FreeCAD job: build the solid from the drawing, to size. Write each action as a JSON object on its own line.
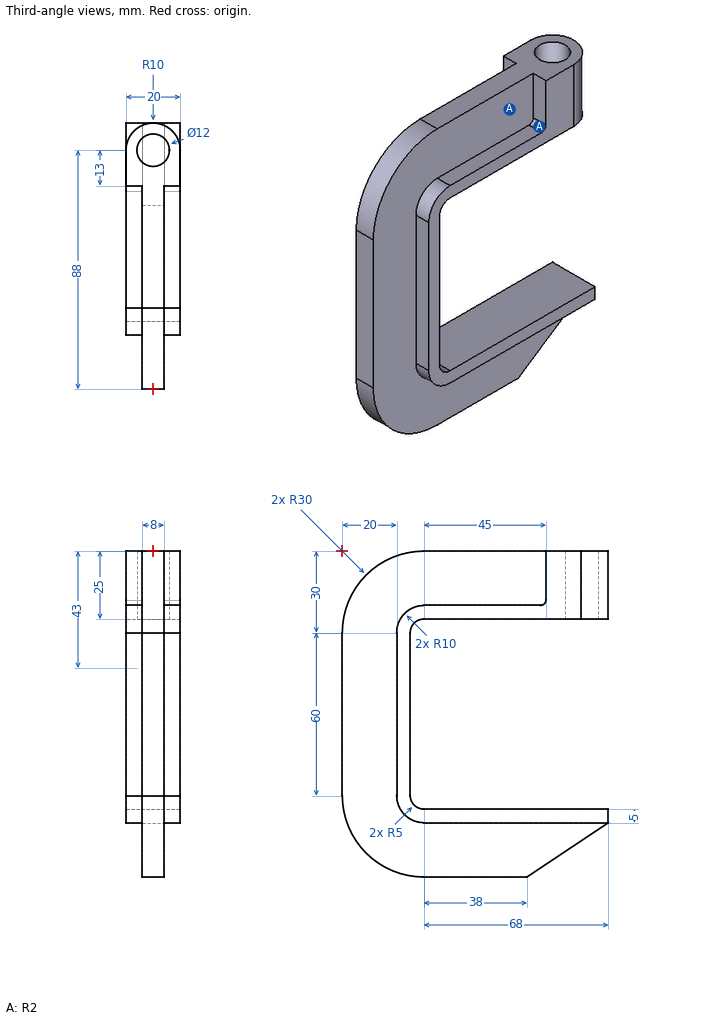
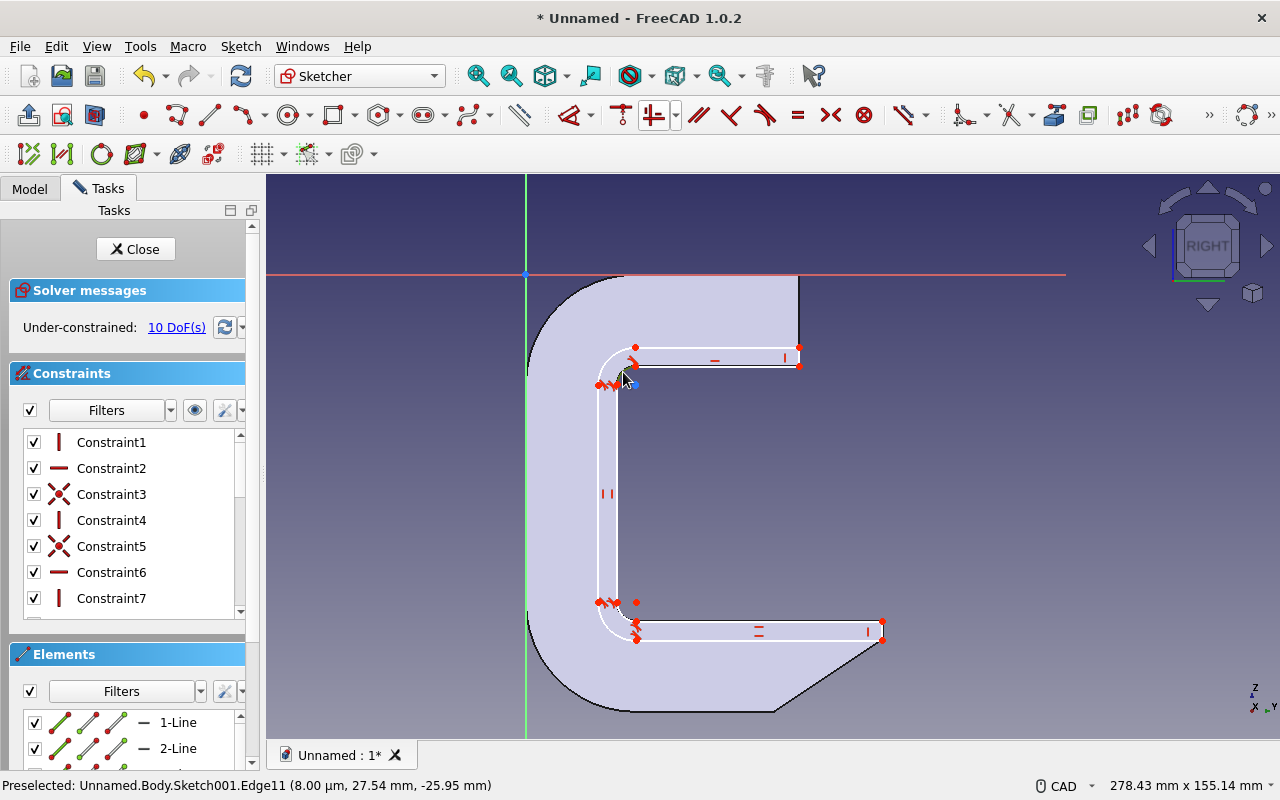
{"action": "left_click", "coordinate": [619, 352]}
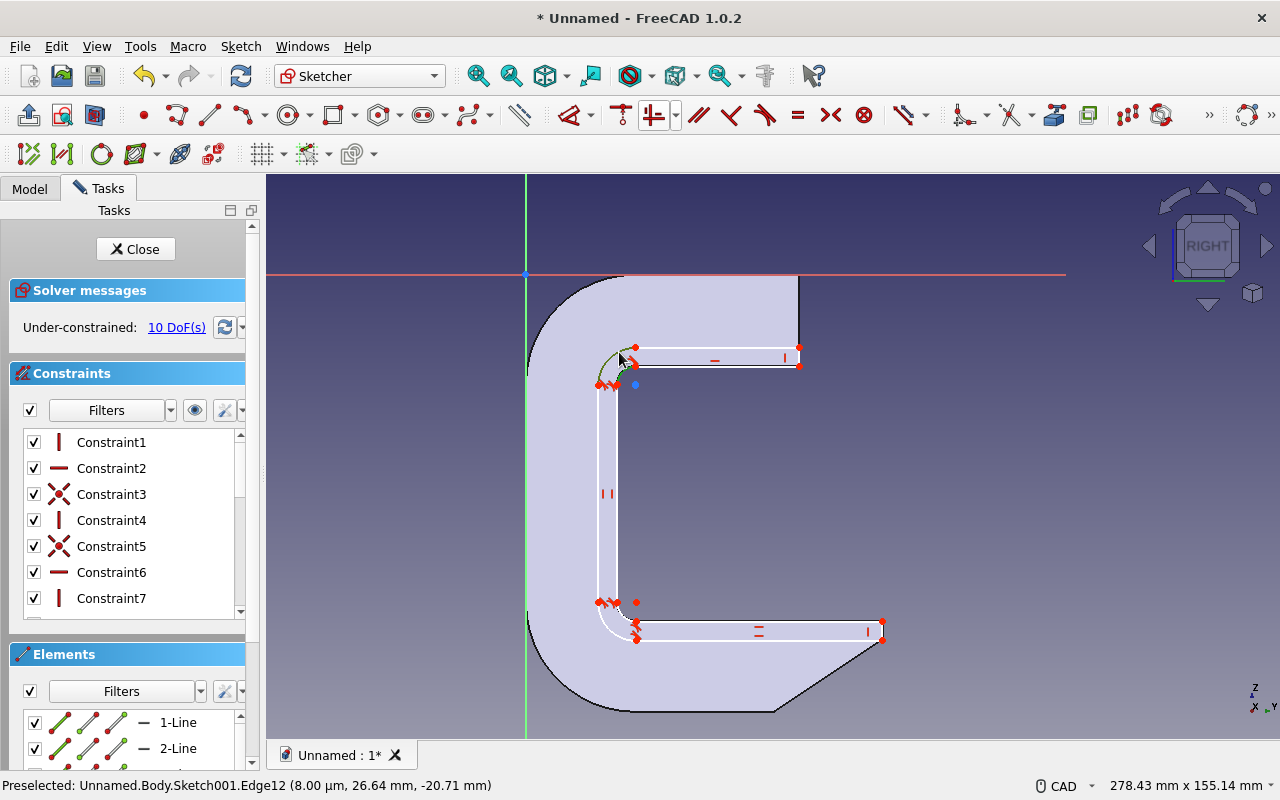
{"action": "key", "text": "c"}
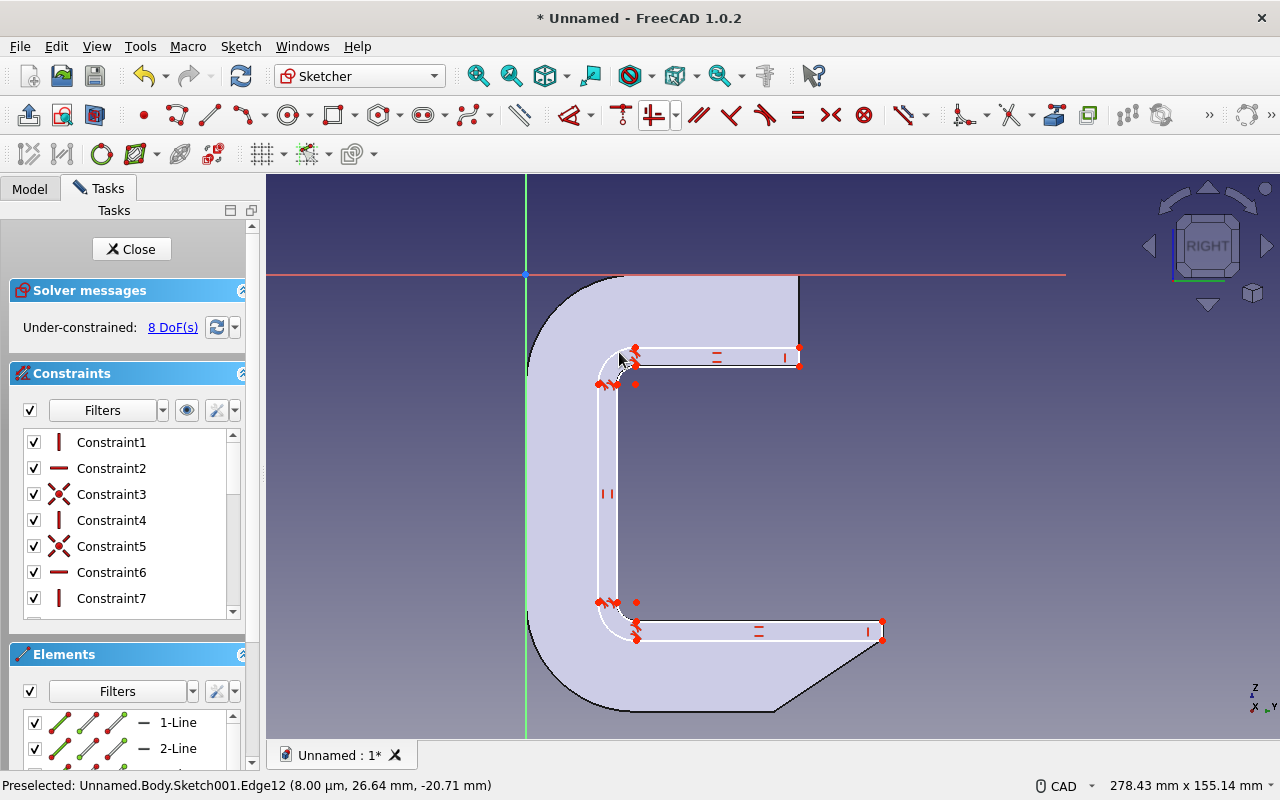
{"action": "left_click", "coordinate": [623, 616]}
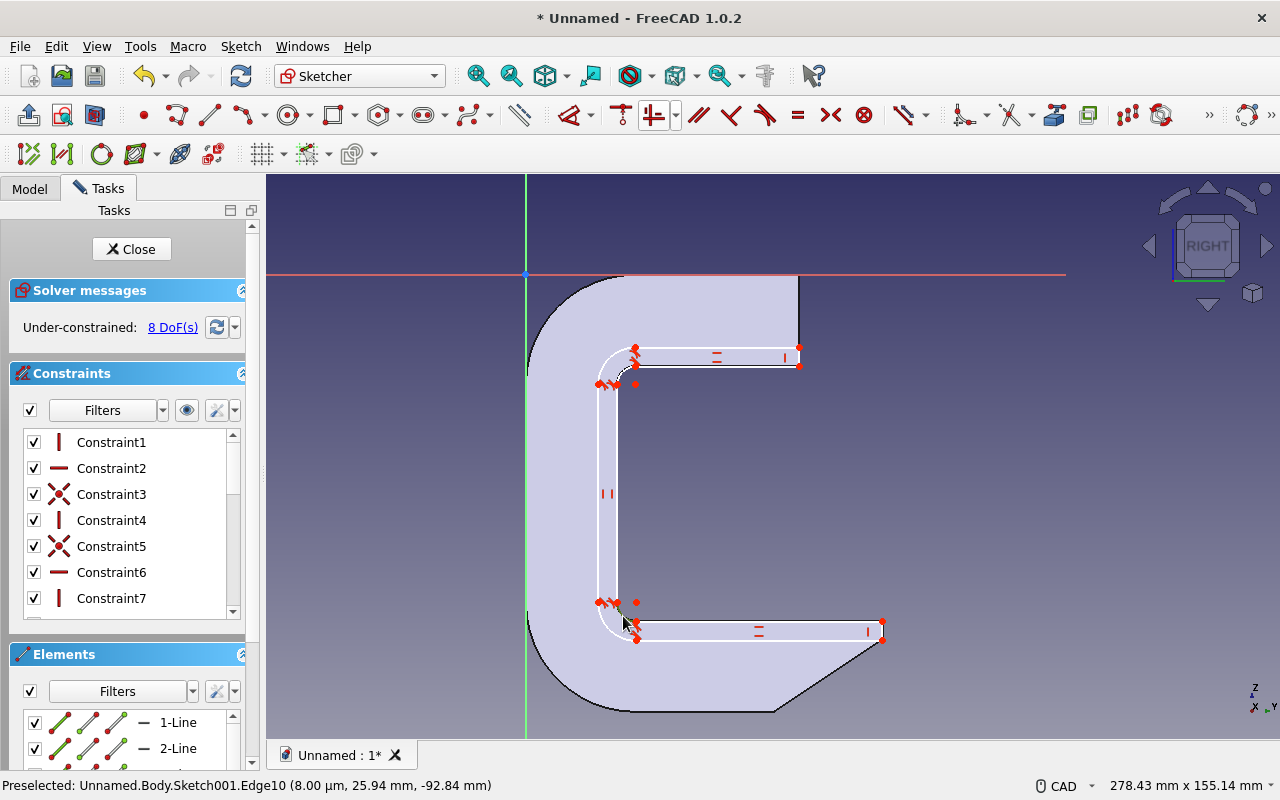
{"action": "left_click", "coordinate": [623, 372]}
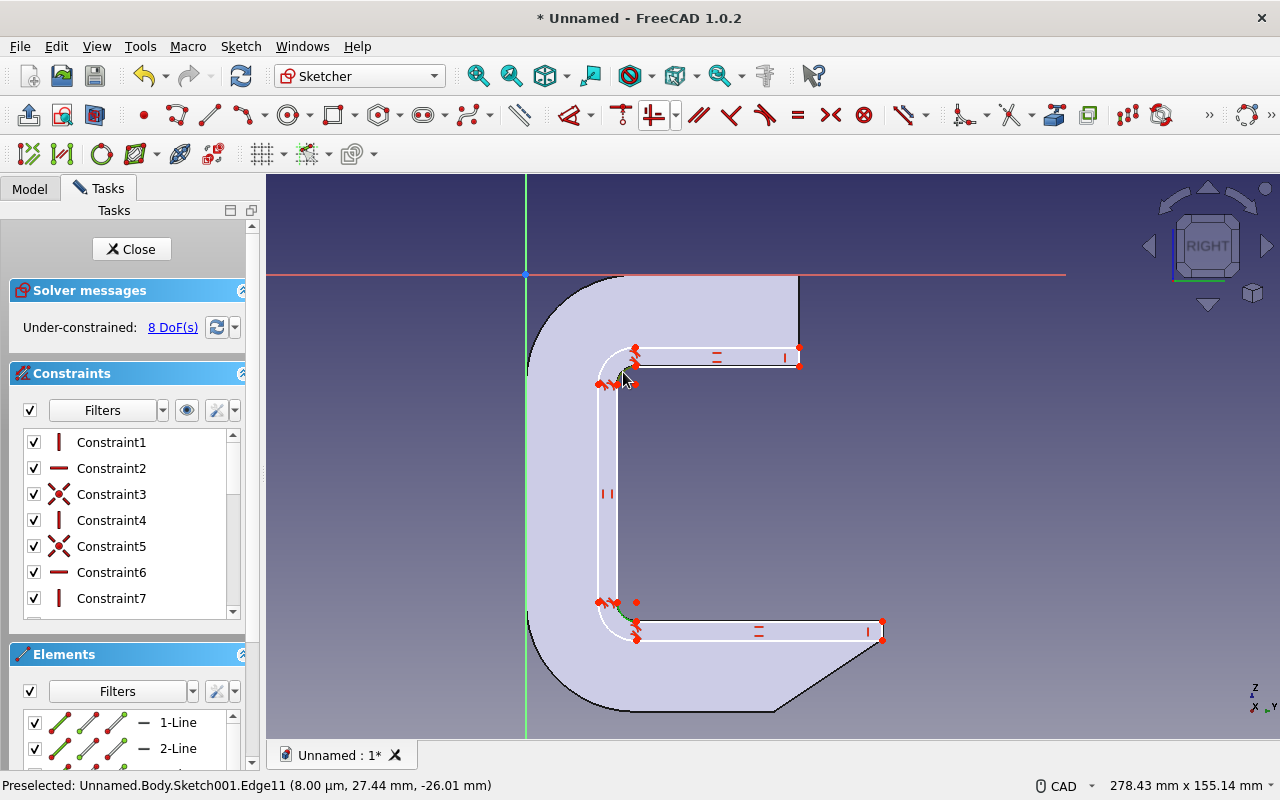
{"action": "key", "text": "e"}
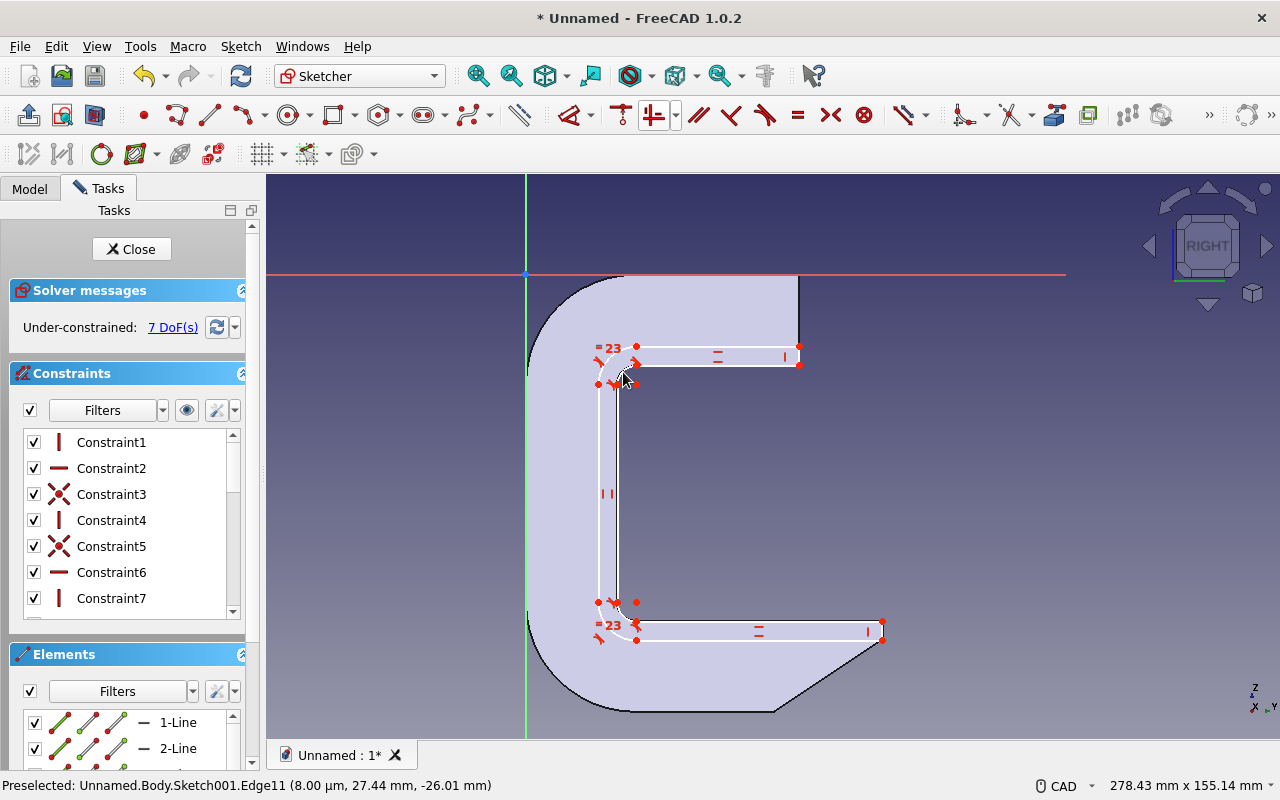
{"action": "key", "text": "d"}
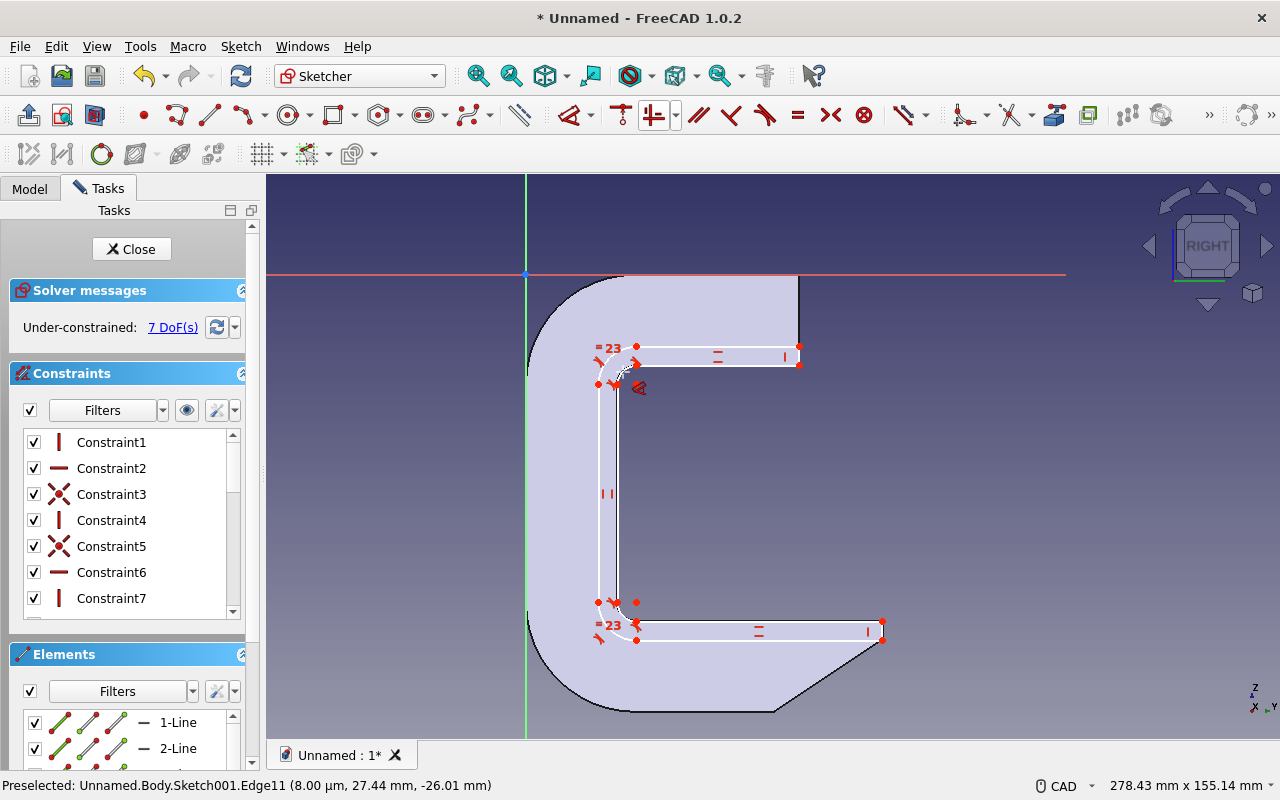
{"action": "left_click", "coordinate": [603, 620]}
{"action": "left_click", "coordinate": [575, 635]}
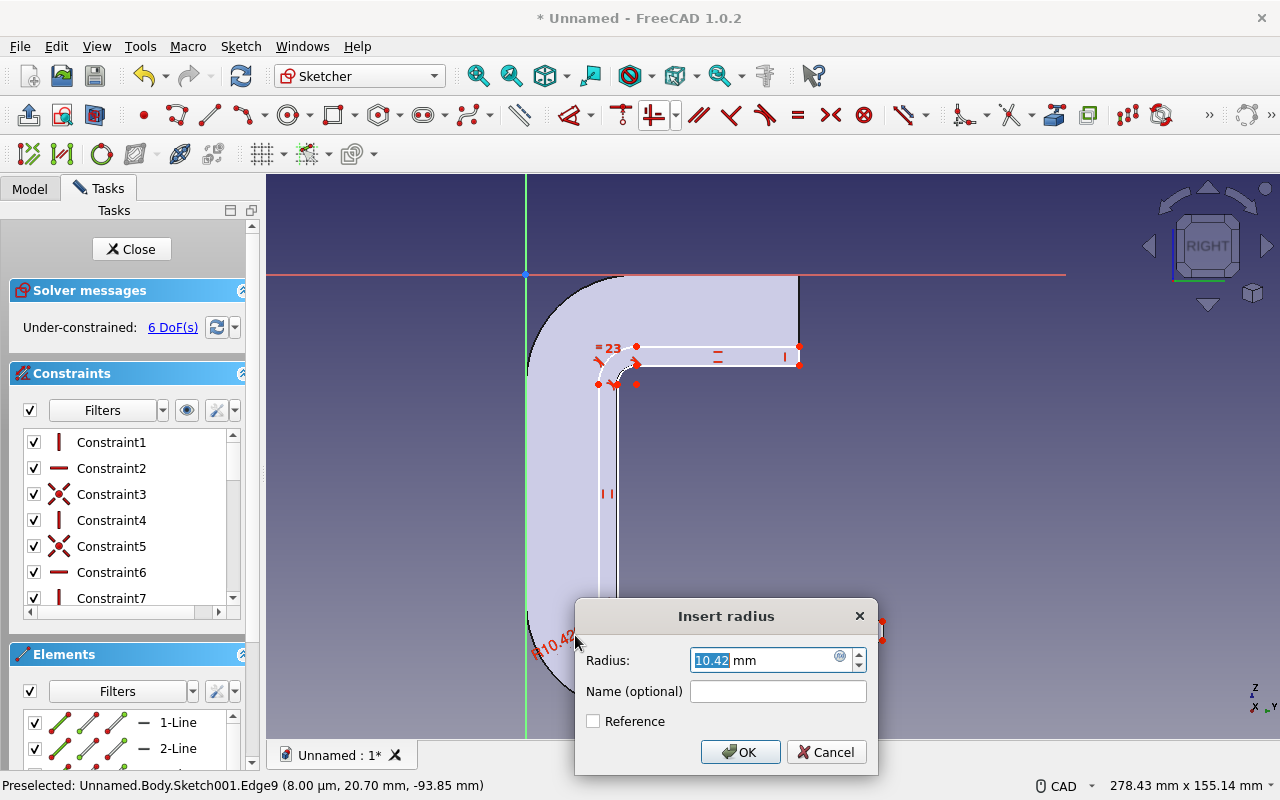
{"action": "type", "text": "10"}
{"action": "key", "text": "Return"}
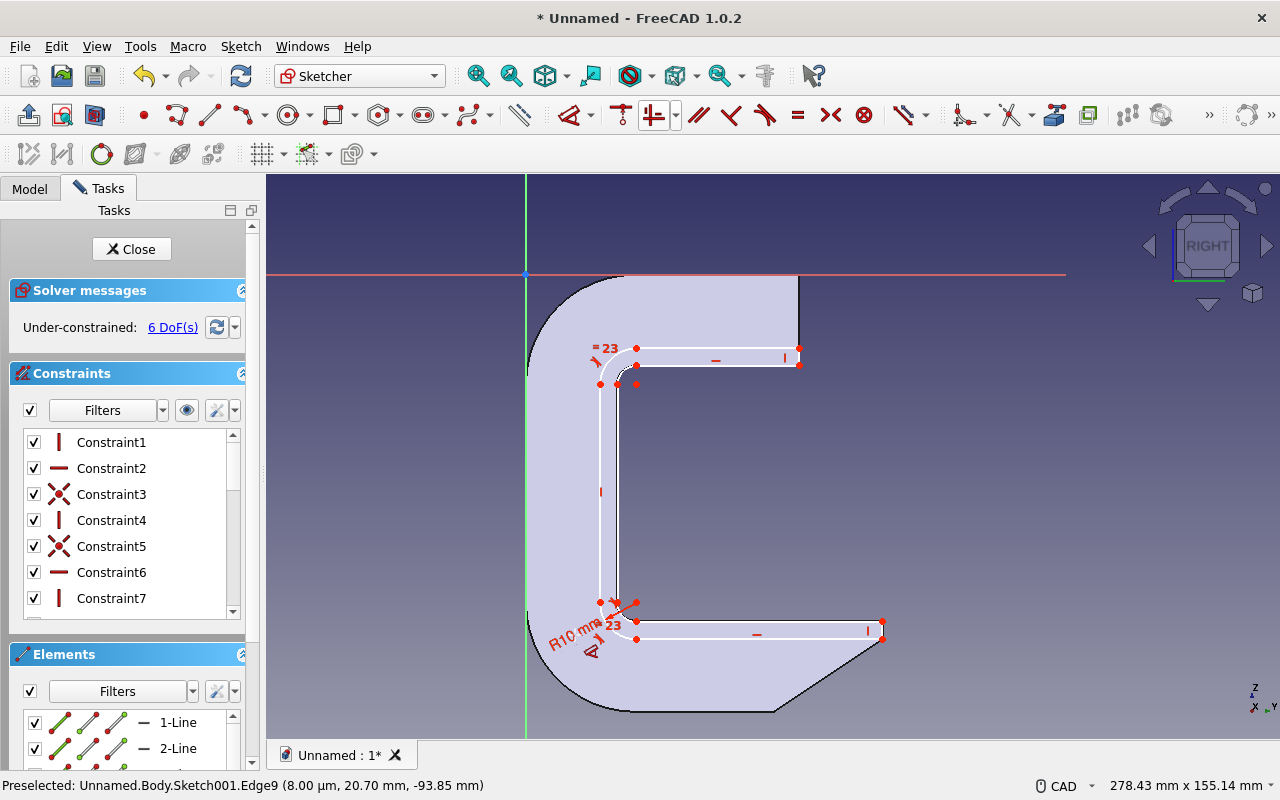
{"action": "scroll", "coordinate": [623, 616], "scroll_direction": "up", "scroll_amount": 4}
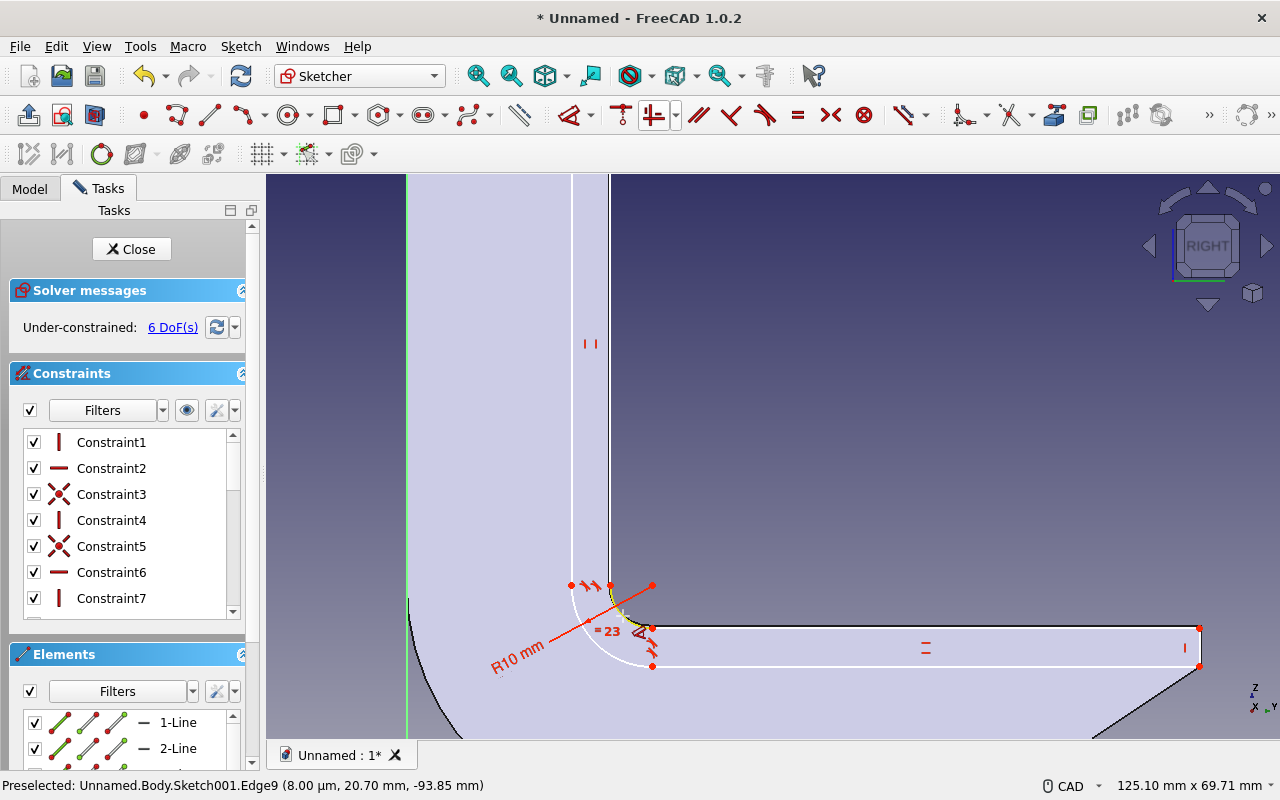
{"action": "left_click", "coordinate": [623, 616]}
{"action": "left_click", "coordinate": [705, 533]}